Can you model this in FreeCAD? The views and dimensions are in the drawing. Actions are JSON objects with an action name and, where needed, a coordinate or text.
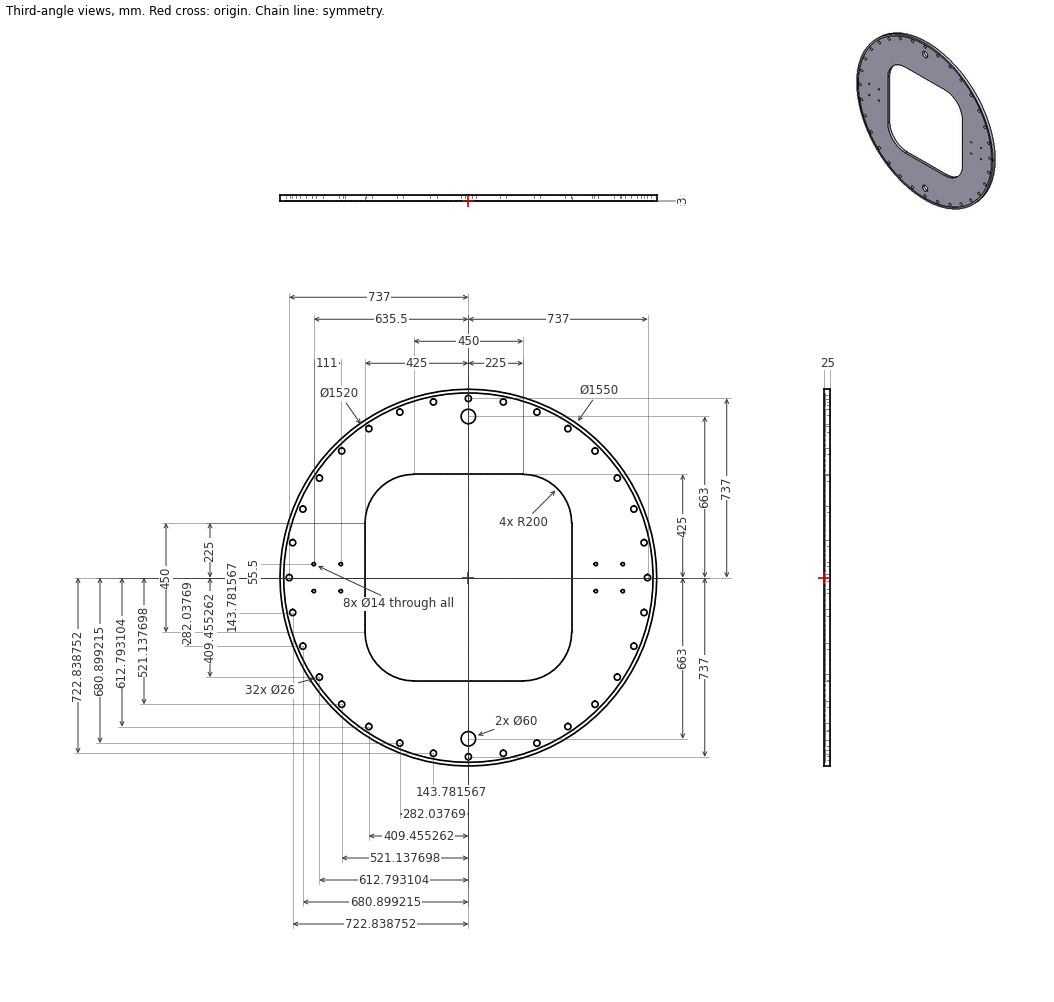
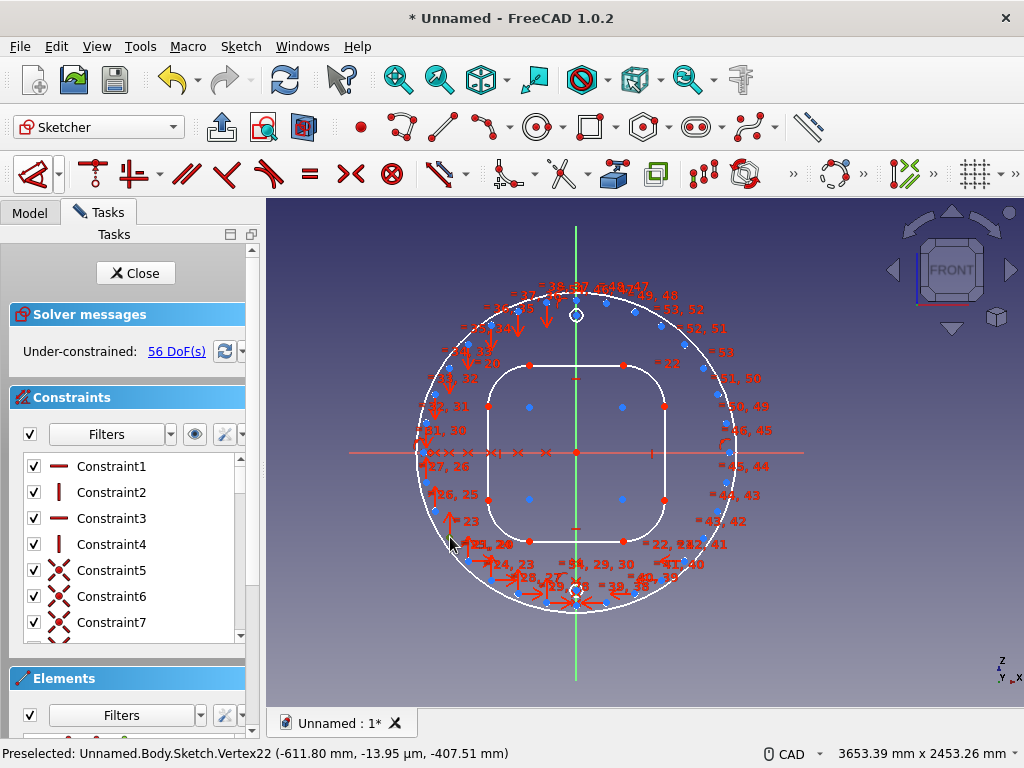
{"action": "left_click", "coordinate": [704, 538]}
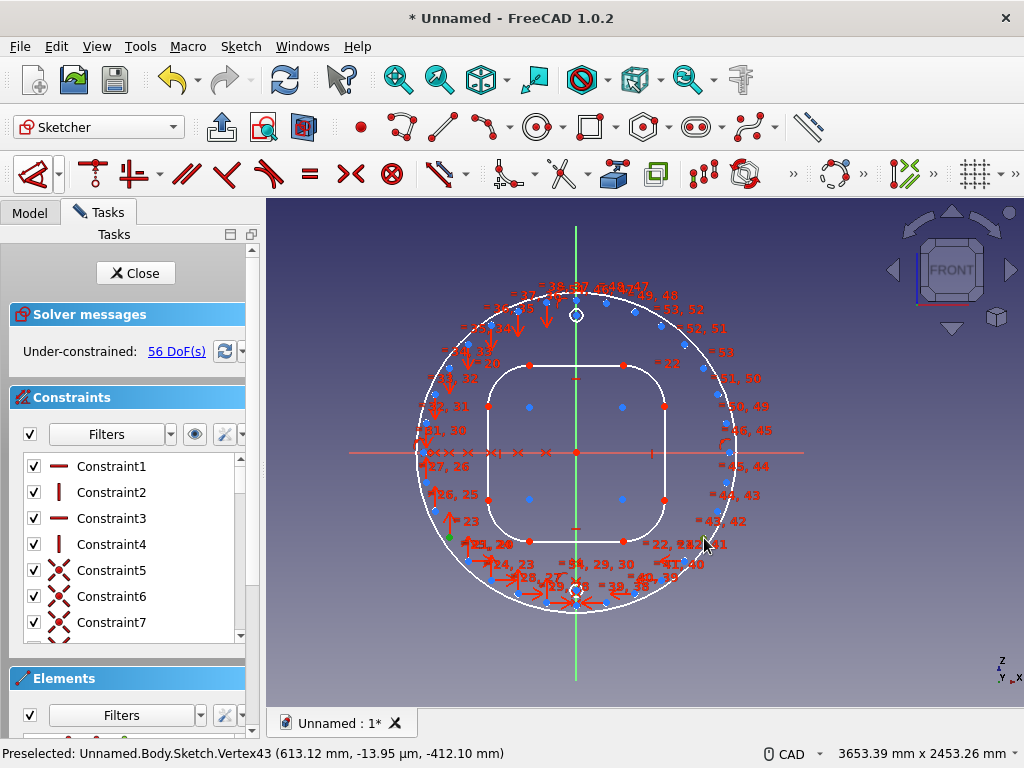
{"action": "left_click", "coordinate": [576, 647]}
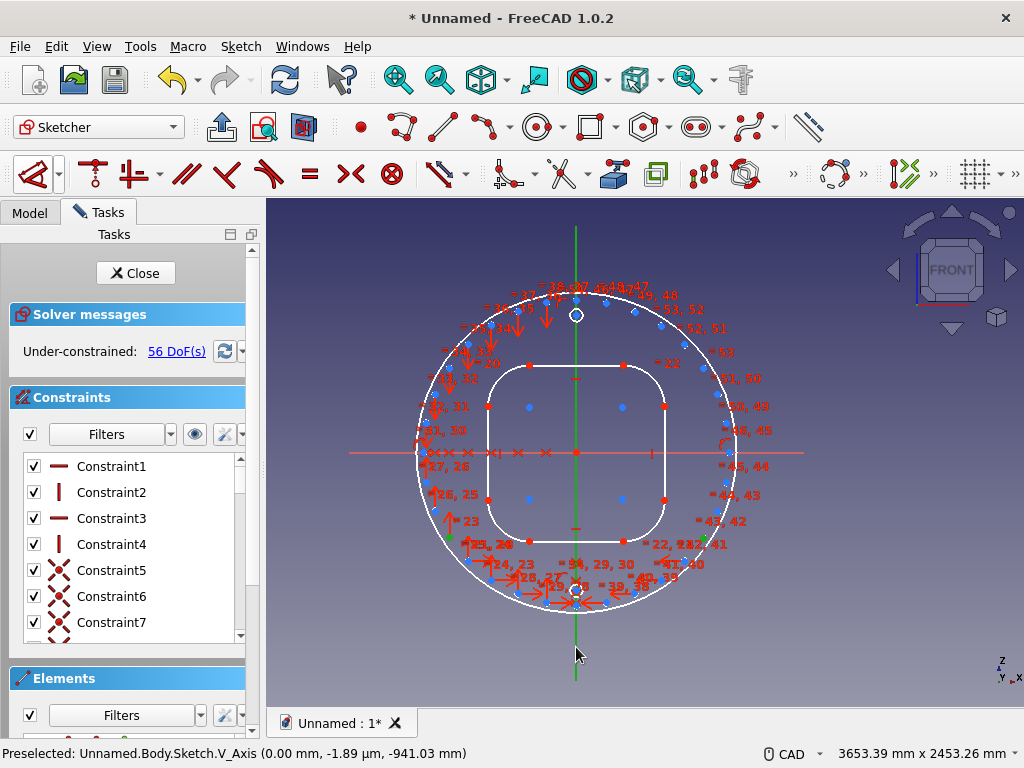
{"action": "left_click", "coordinate": [351, 174]}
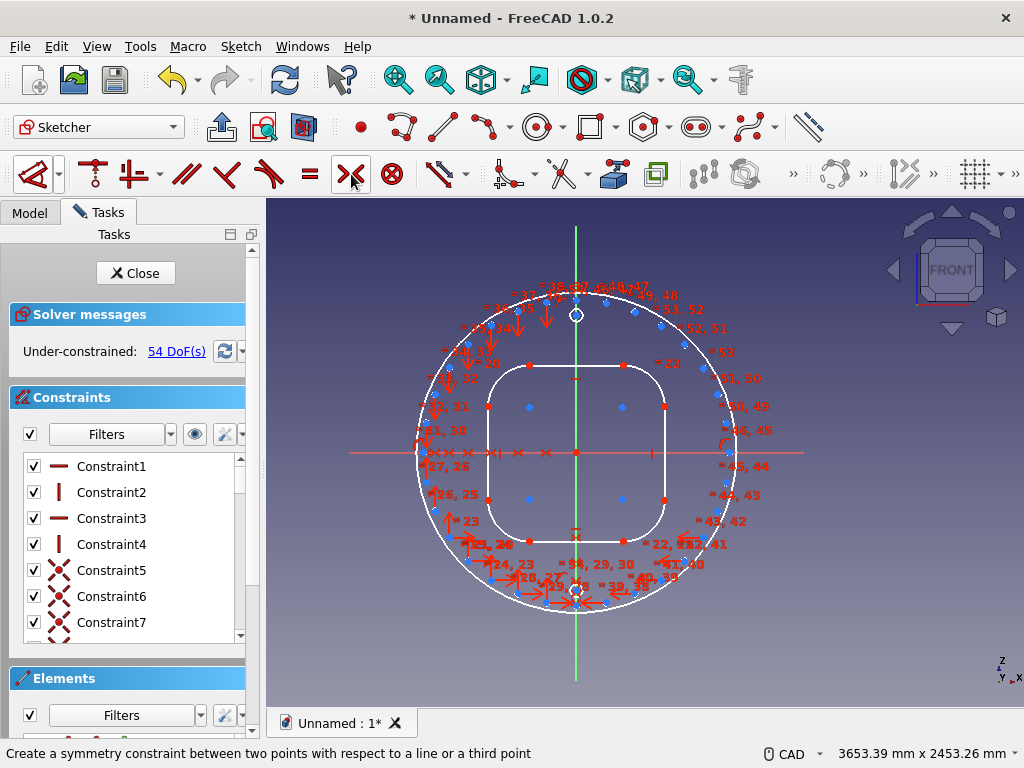
{"action": "left_click", "coordinate": [435, 511]}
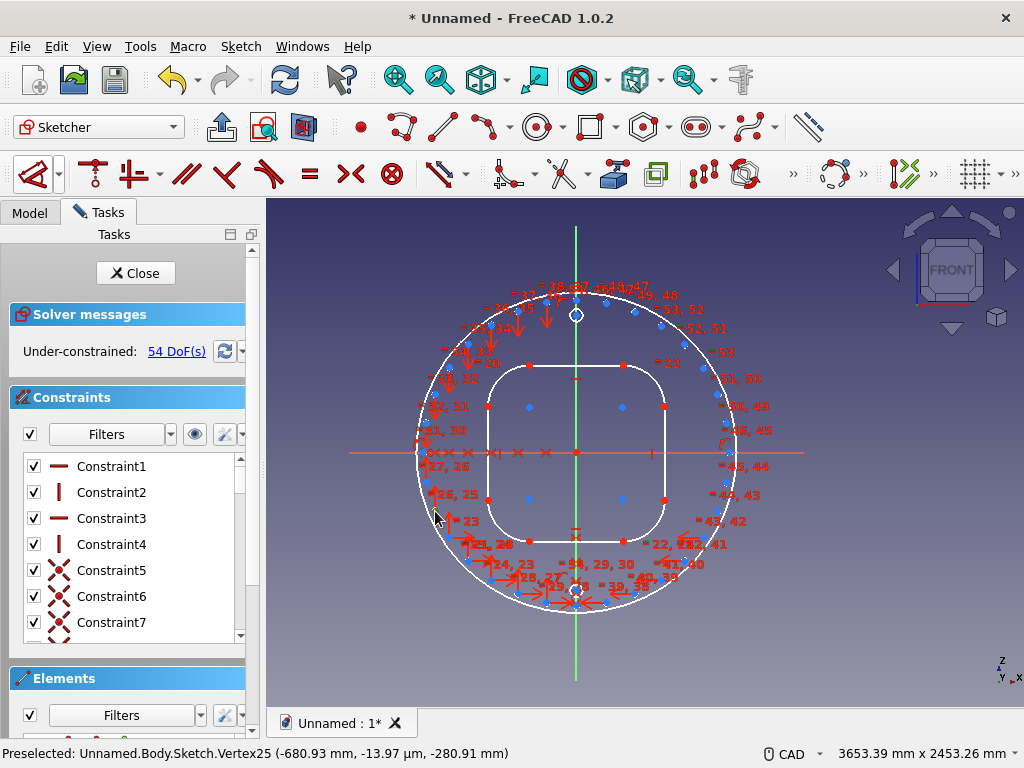
{"action": "left_click", "coordinate": [718, 512]}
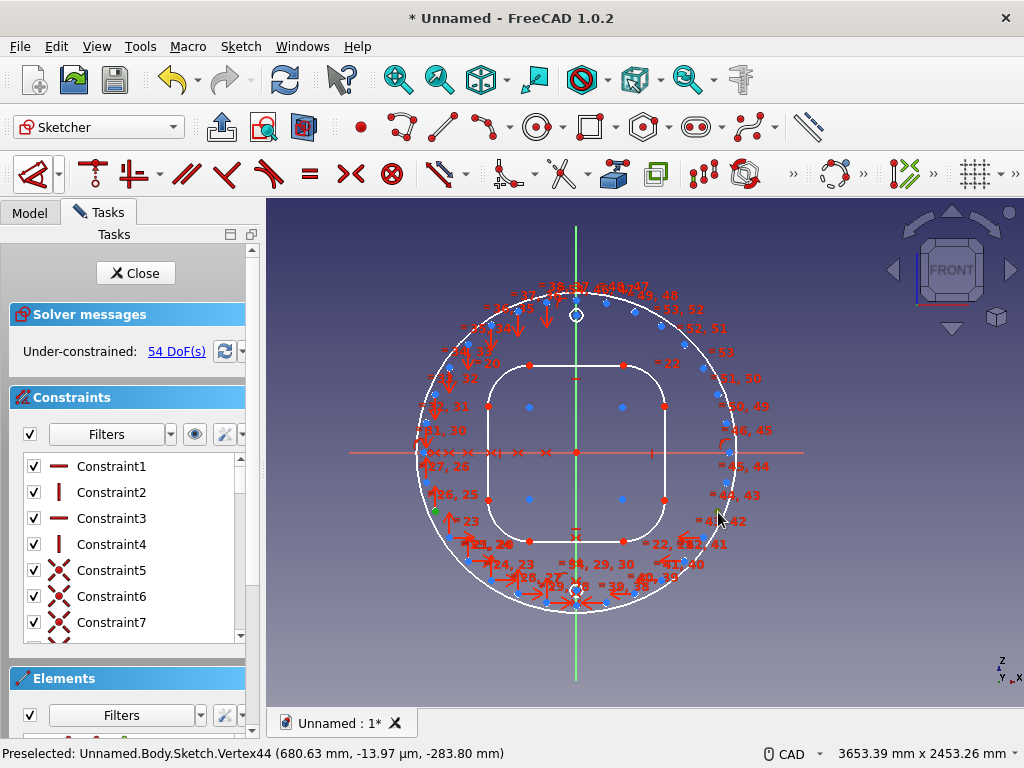
{"action": "left_click", "coordinate": [576, 647]}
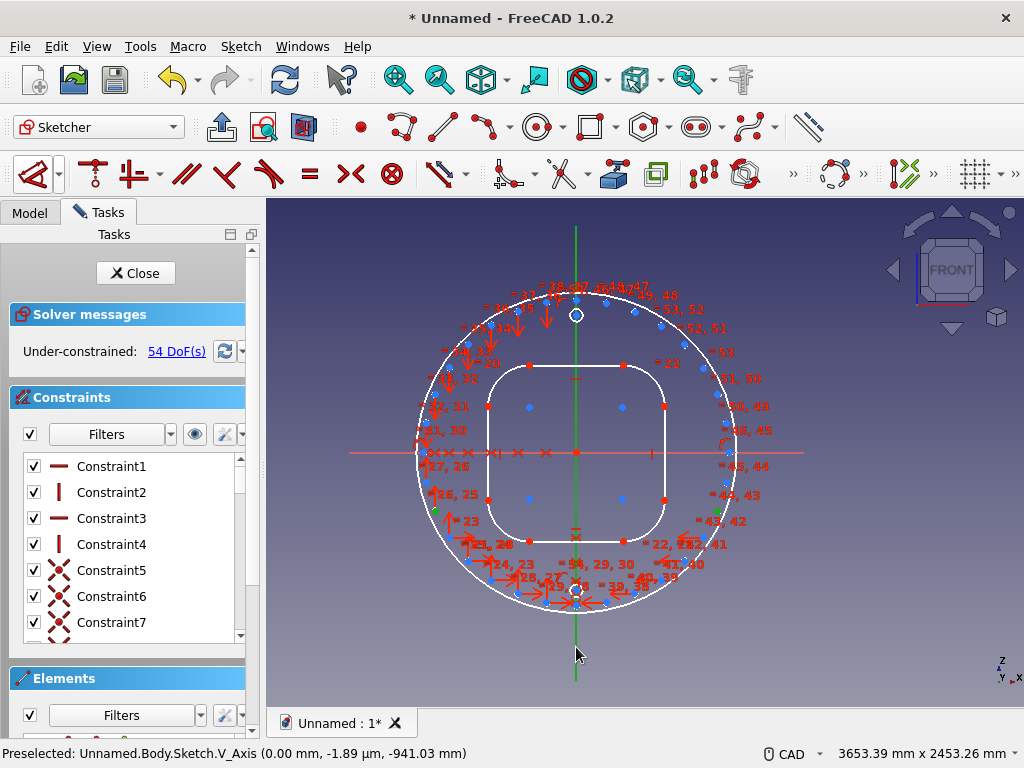
{"action": "left_click", "coordinate": [351, 174]}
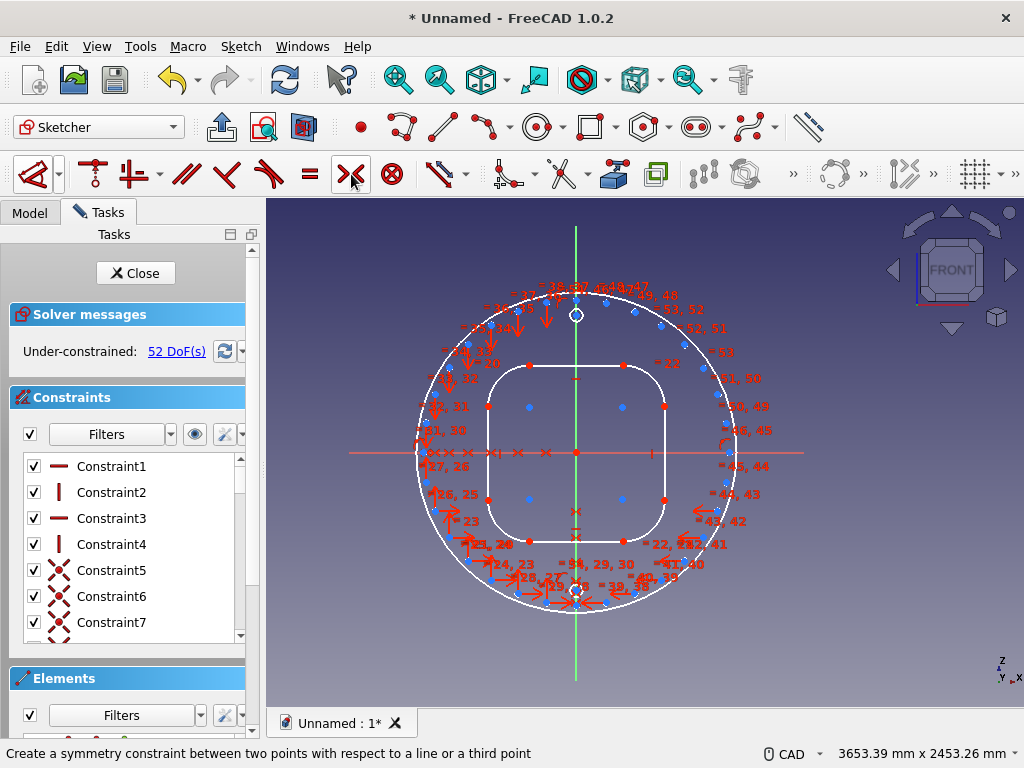
{"action": "left_click", "coordinate": [426, 483]}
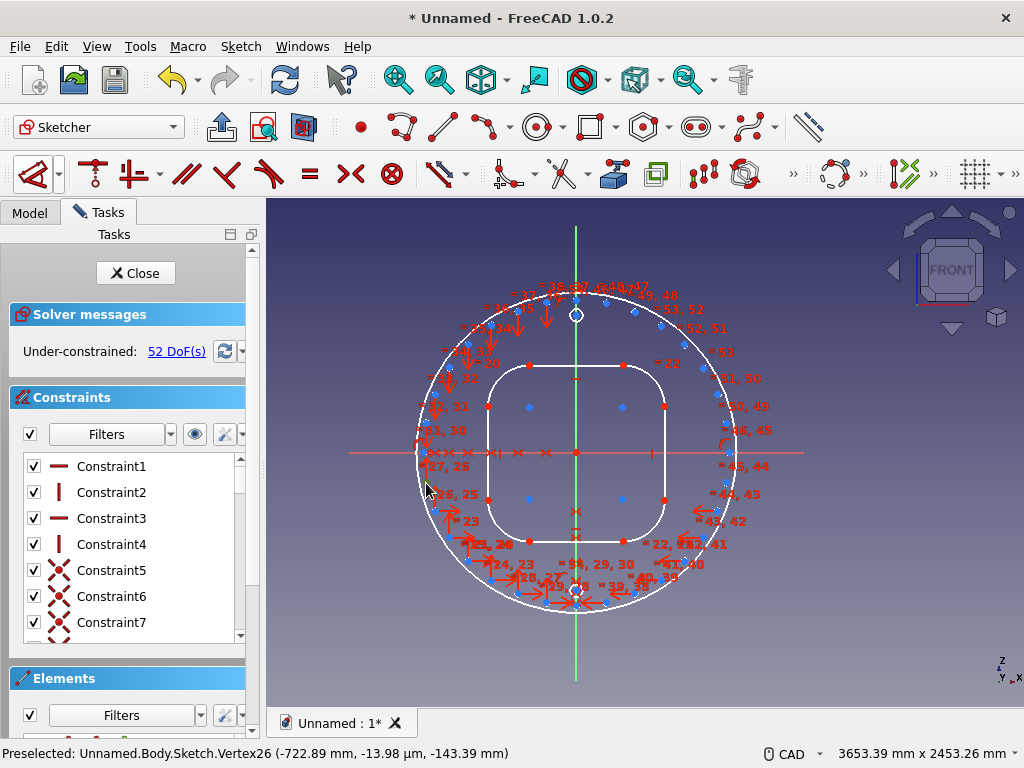
{"action": "left_click", "coordinate": [726, 483]}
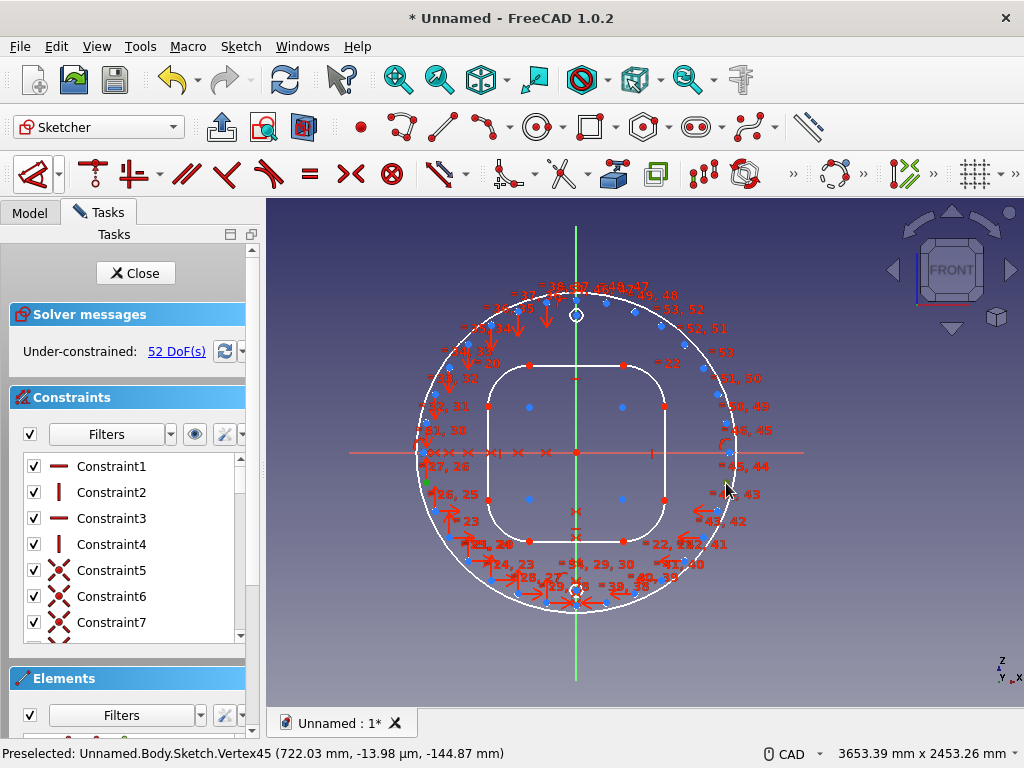
{"action": "left_click", "coordinate": [576, 647]}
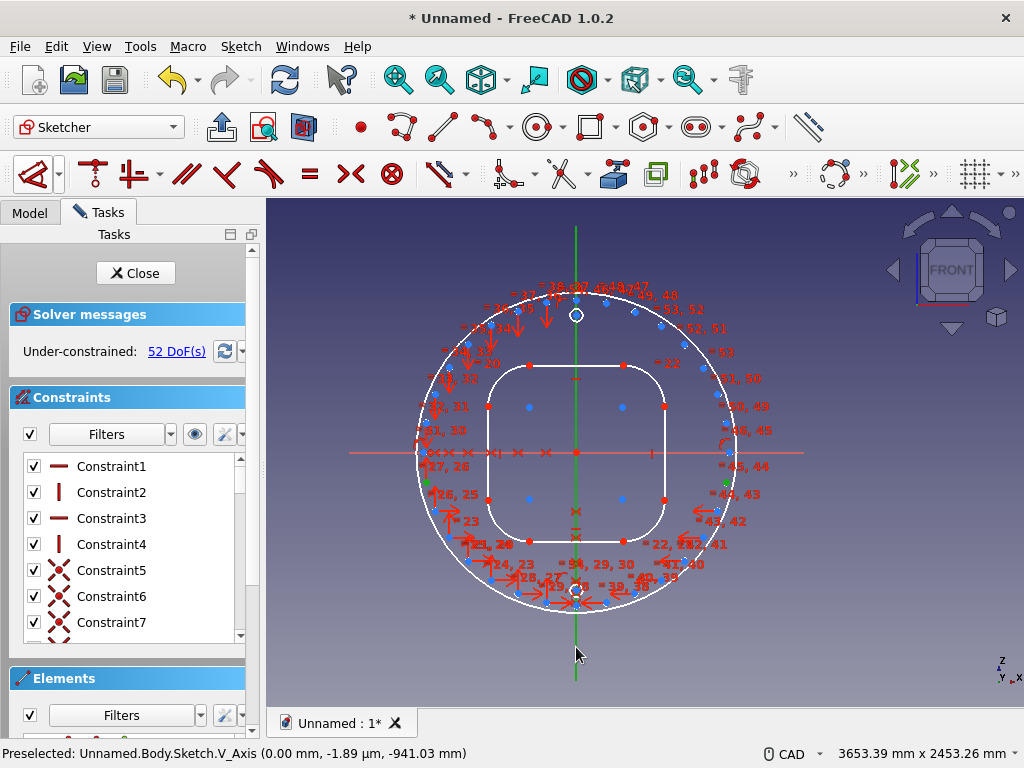
{"action": "left_click", "coordinate": [351, 174]}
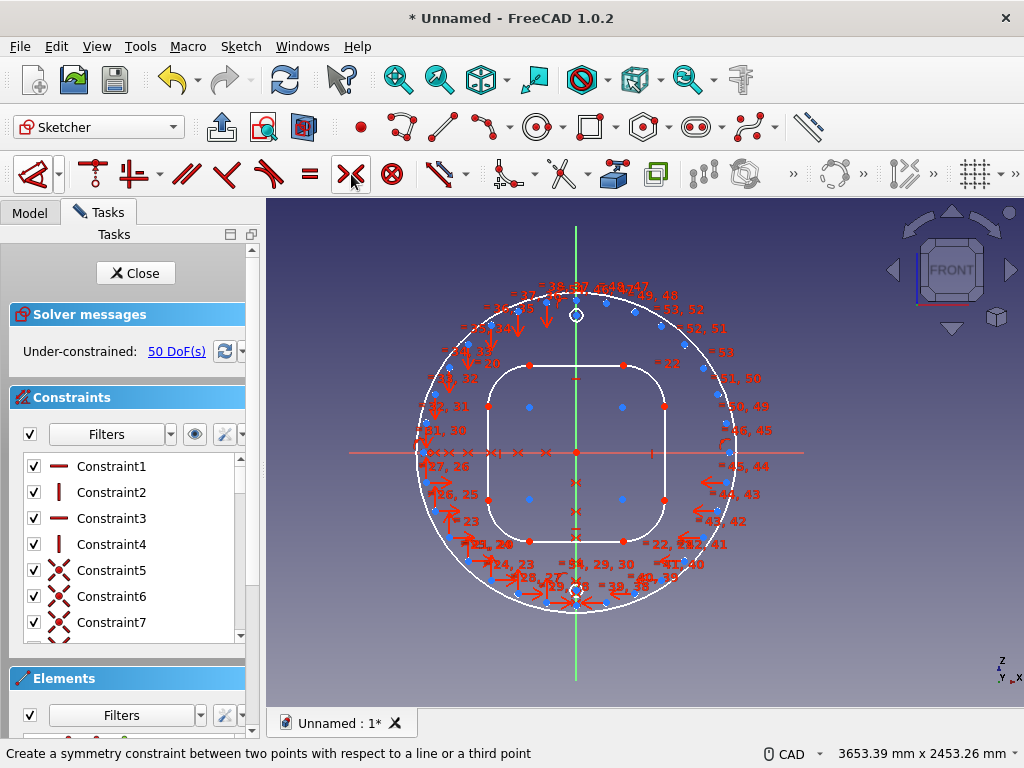
{"action": "left_click", "coordinate": [547, 303]}